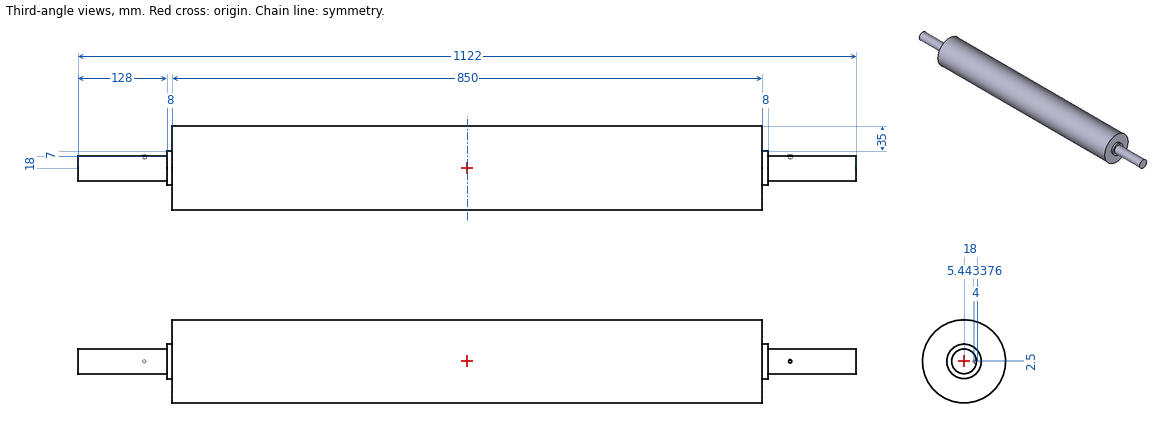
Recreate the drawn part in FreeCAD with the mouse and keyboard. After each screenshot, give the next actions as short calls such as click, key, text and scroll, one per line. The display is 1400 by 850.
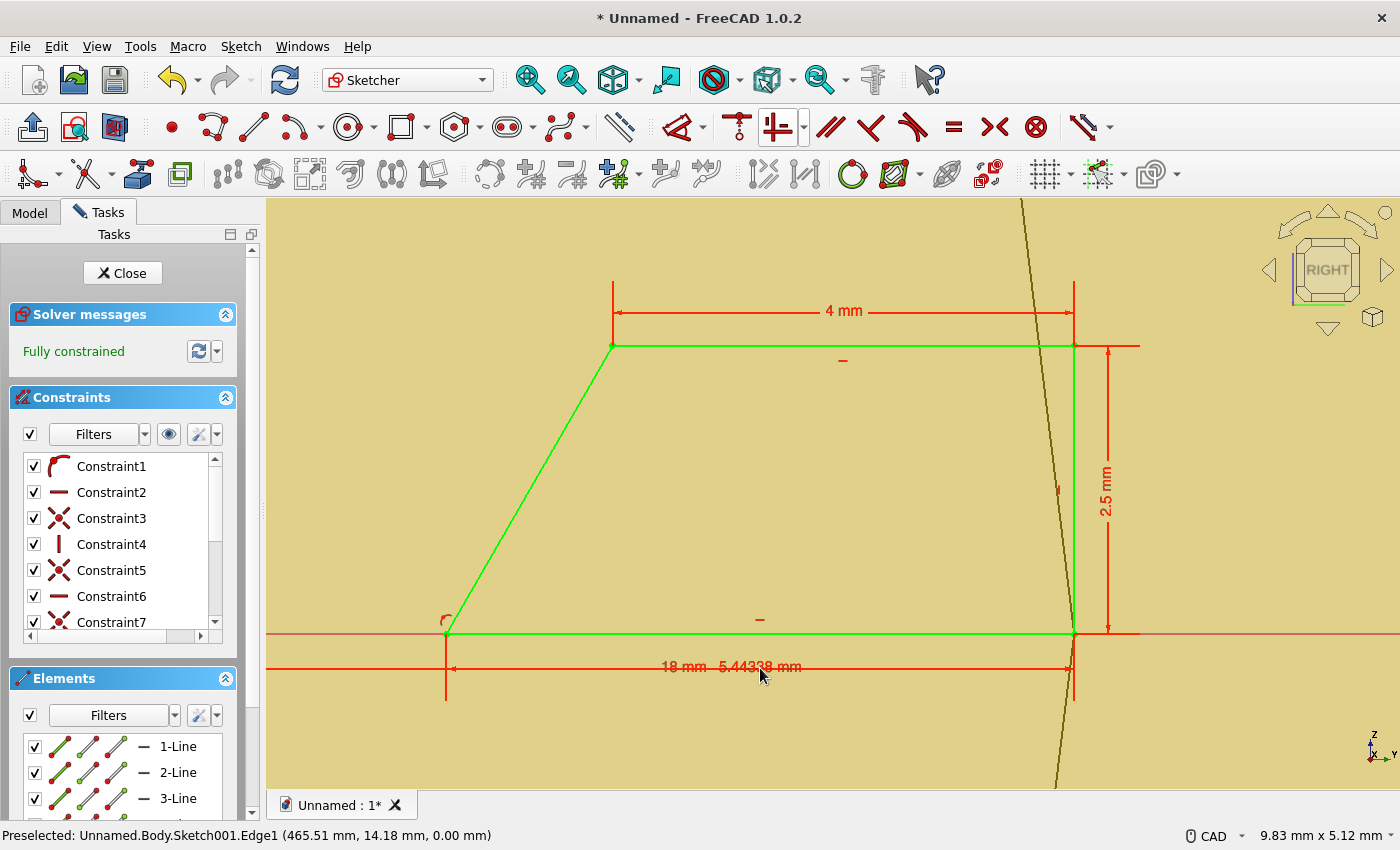
click(123, 273)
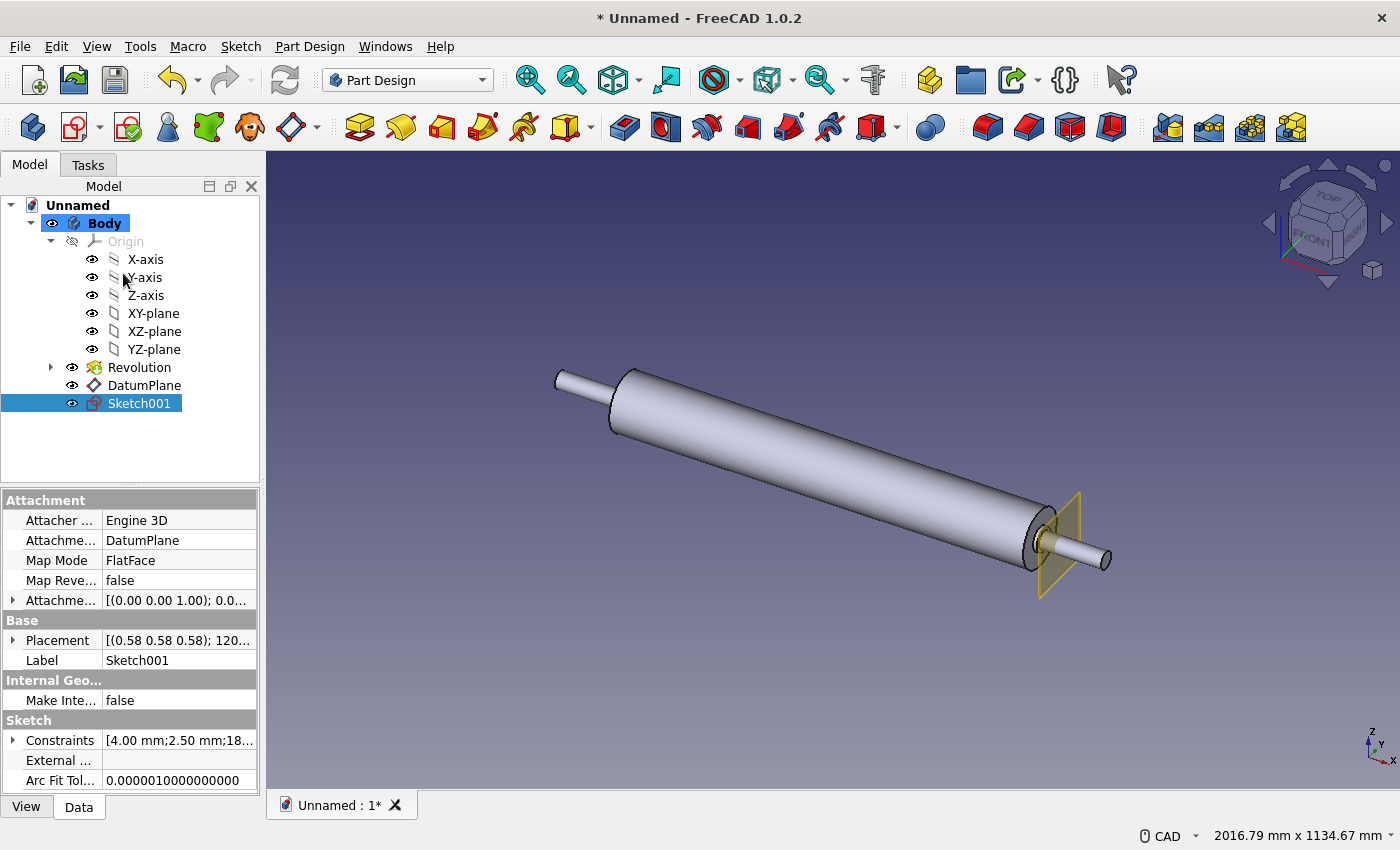
click(707, 128)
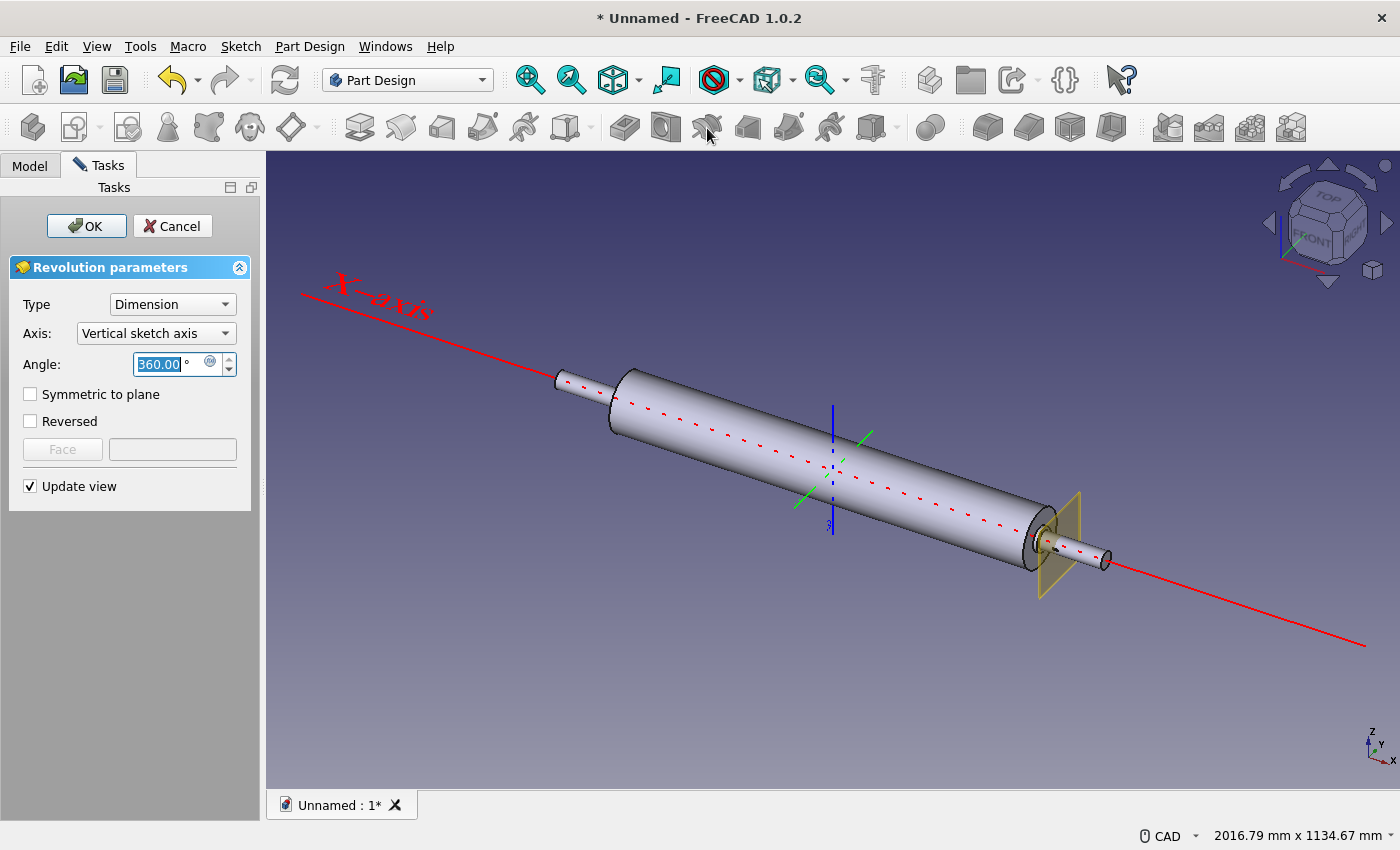
click(157, 334)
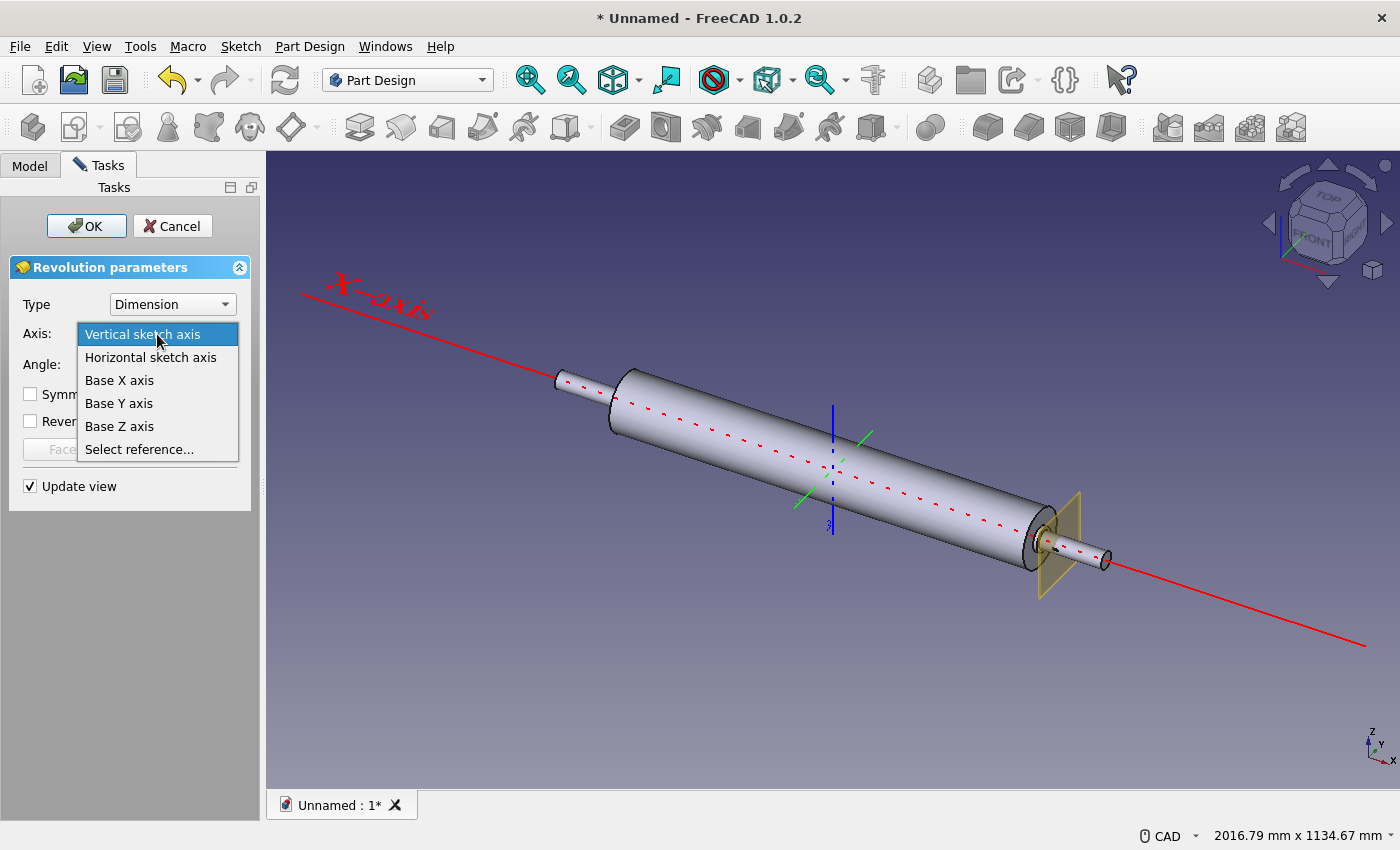
click(156, 358)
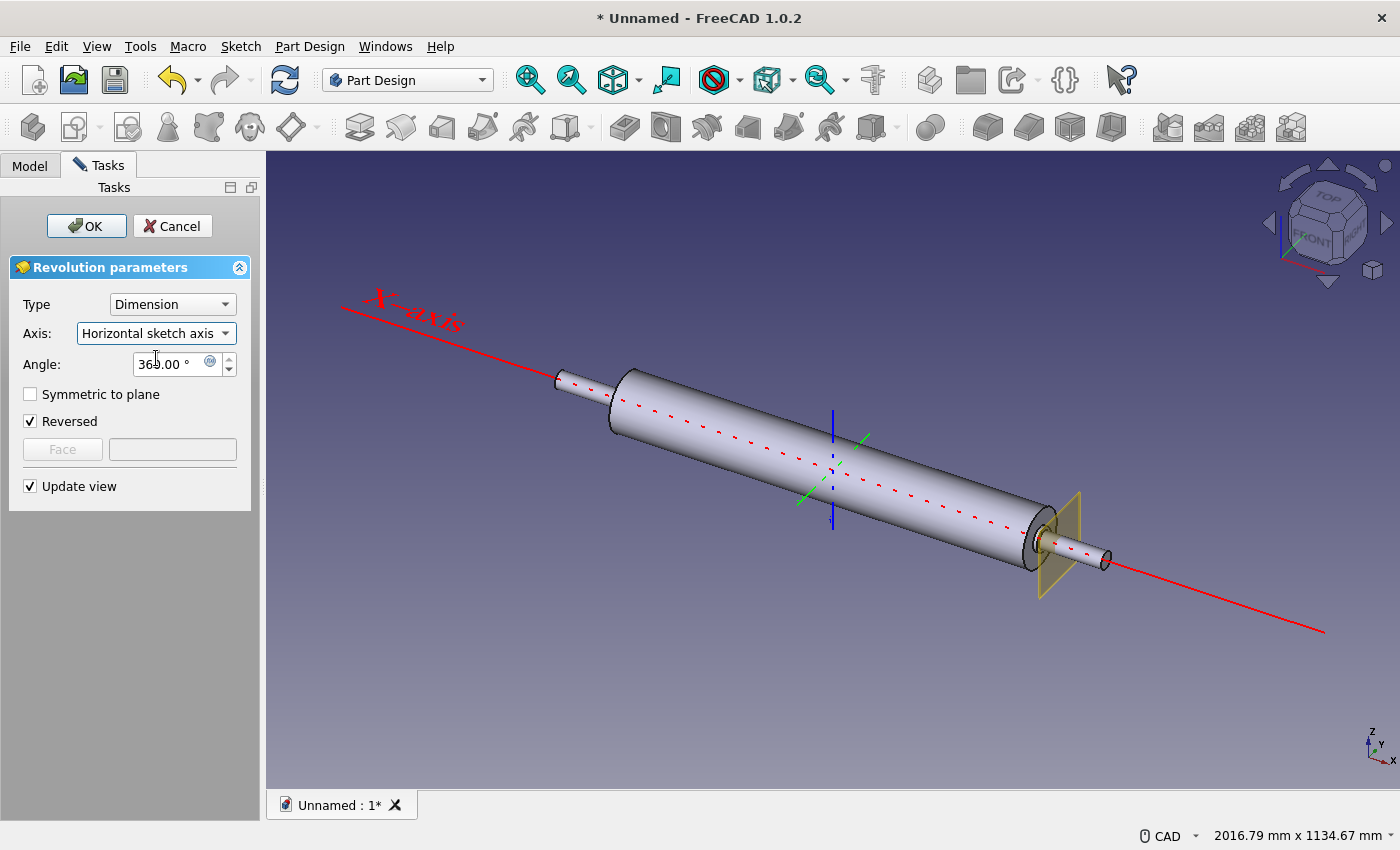
click(87, 226)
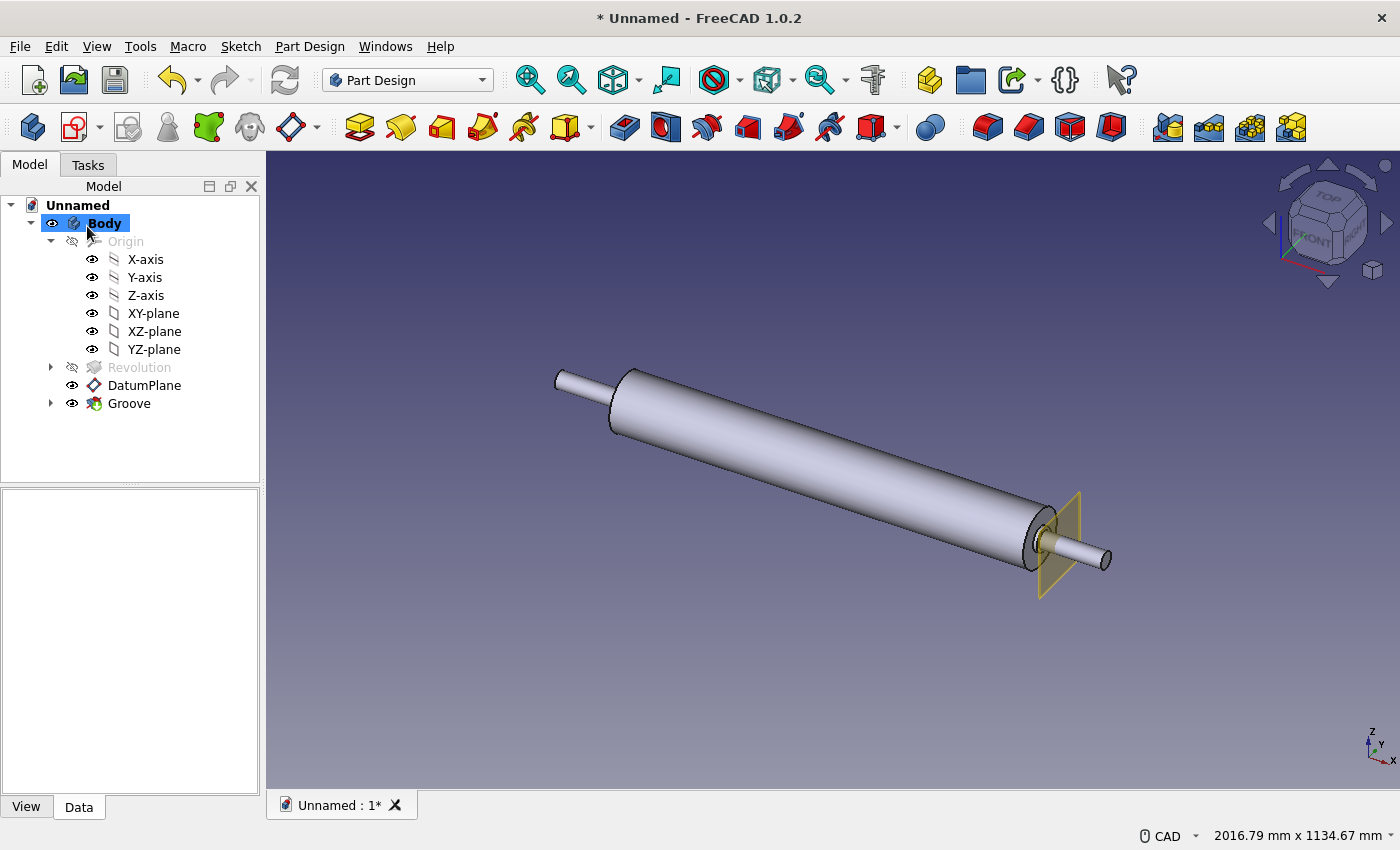
click(117, 385)
key(space)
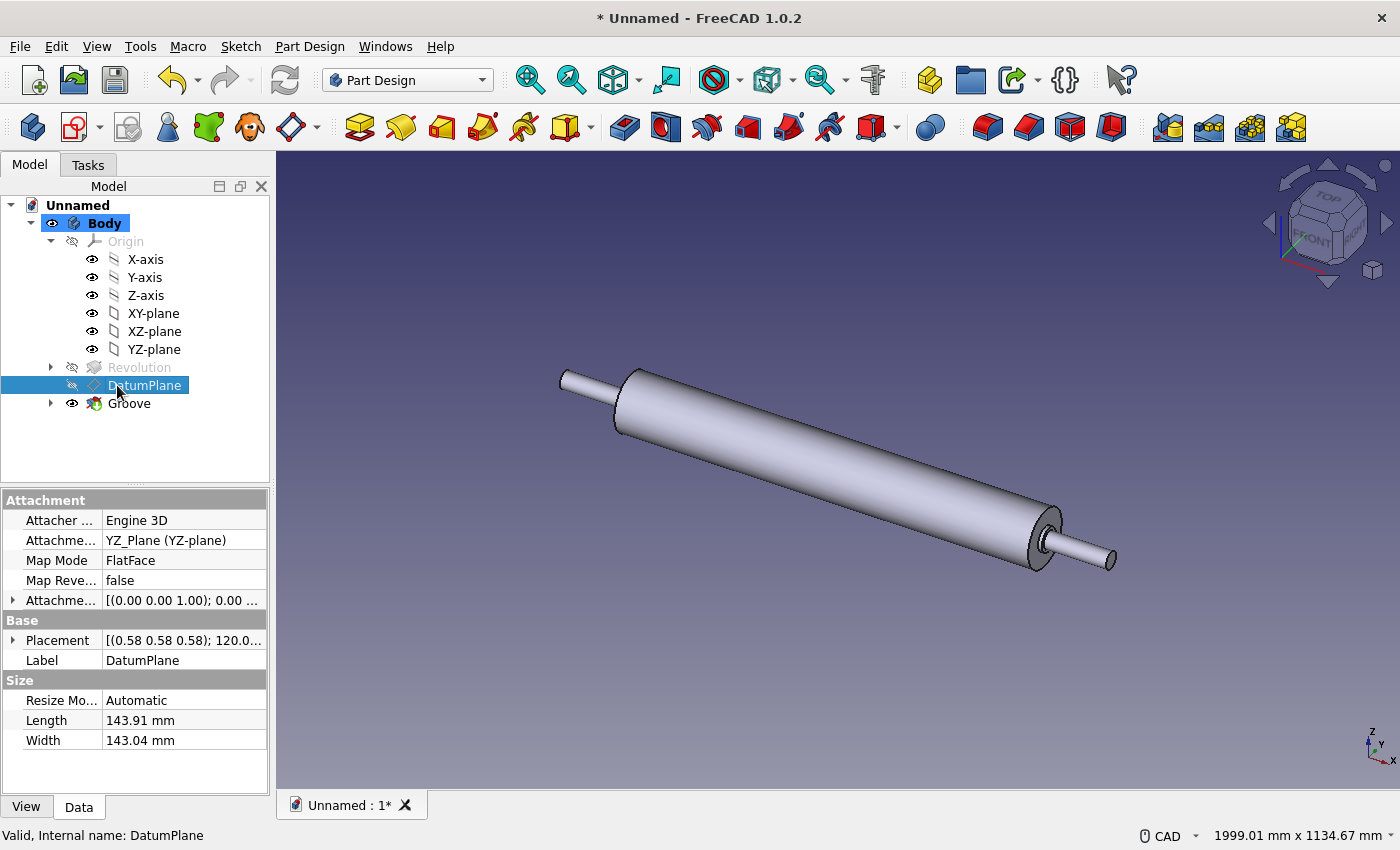
click(117, 403)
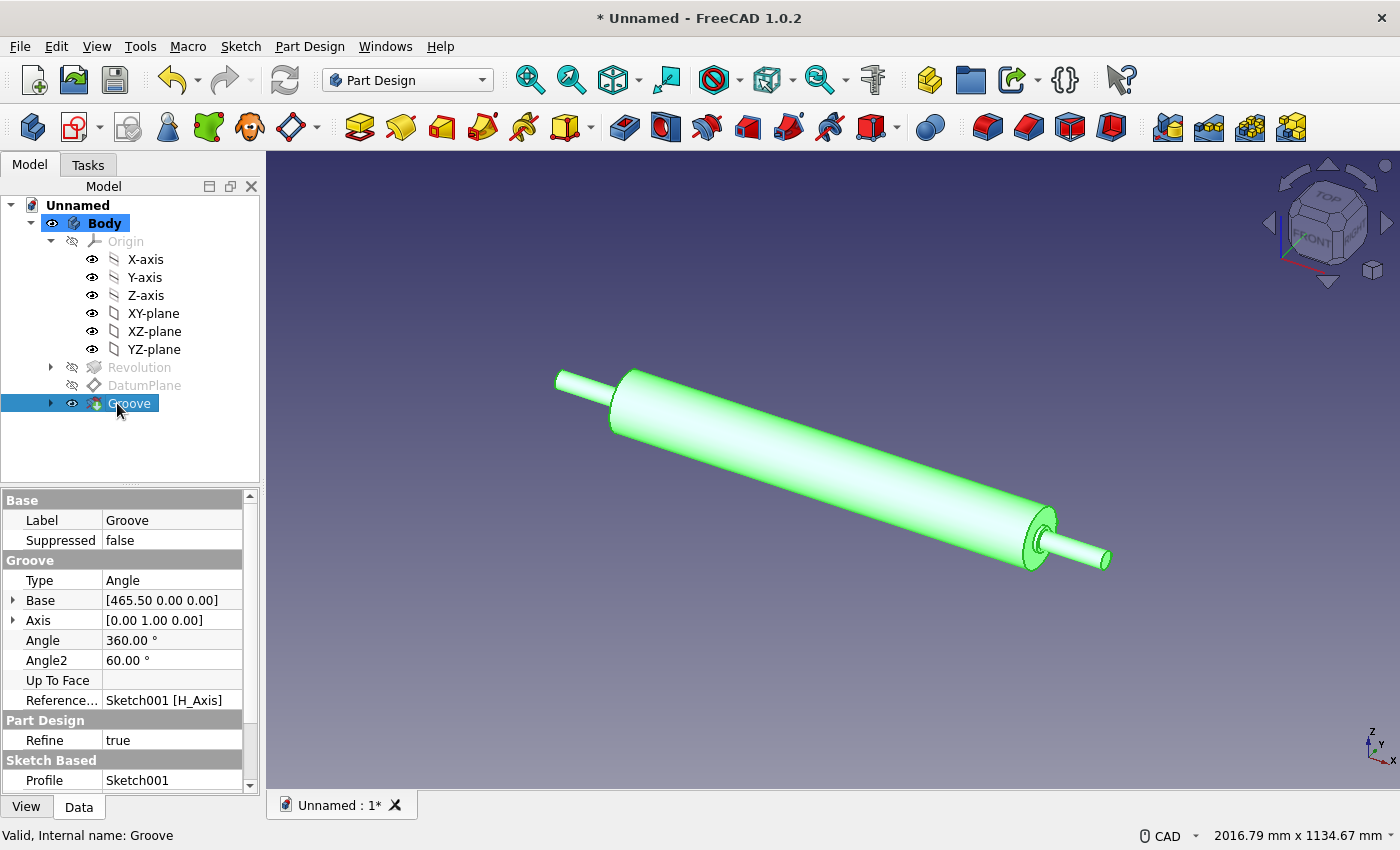
click(1168, 128)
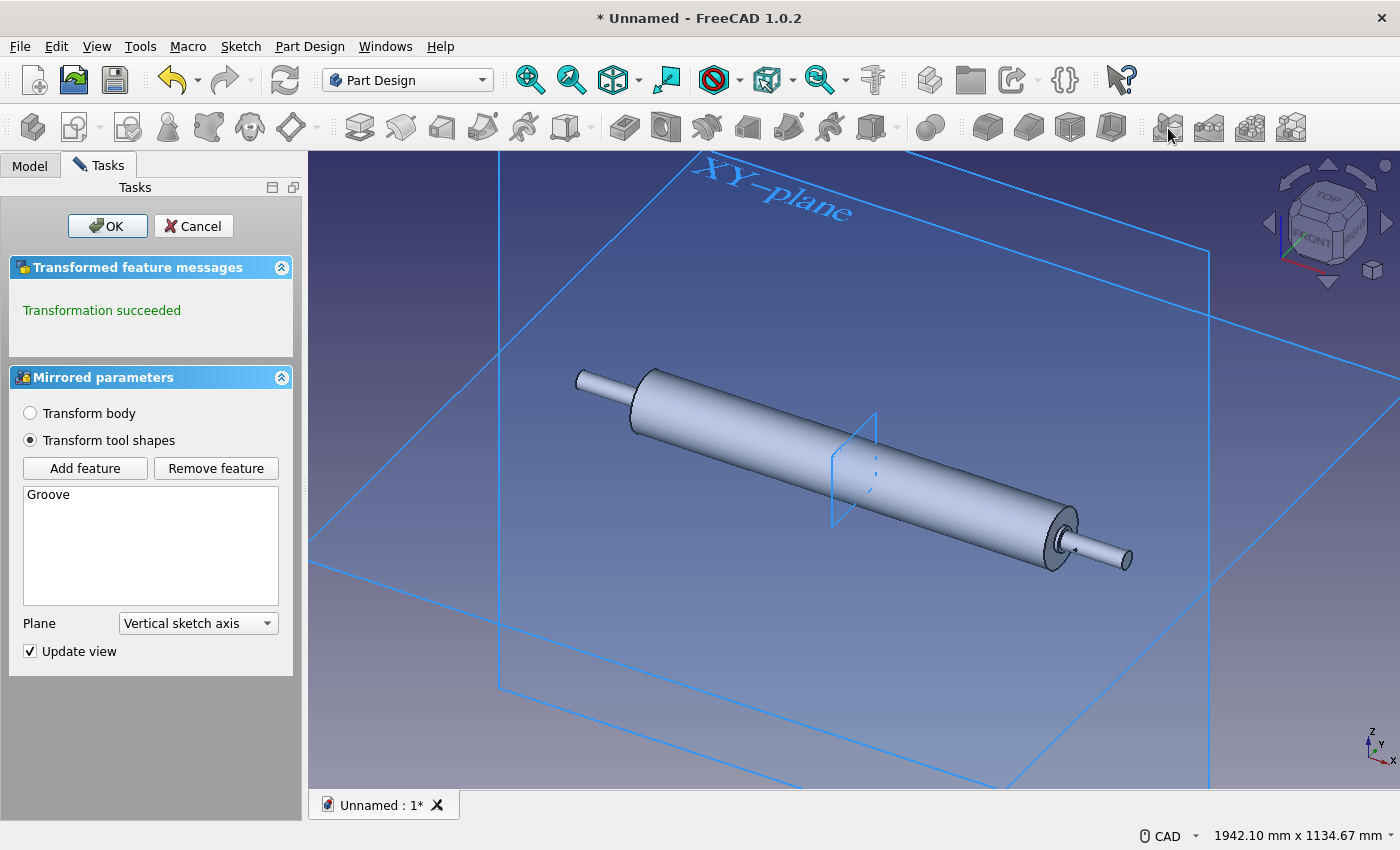
click(199, 624)